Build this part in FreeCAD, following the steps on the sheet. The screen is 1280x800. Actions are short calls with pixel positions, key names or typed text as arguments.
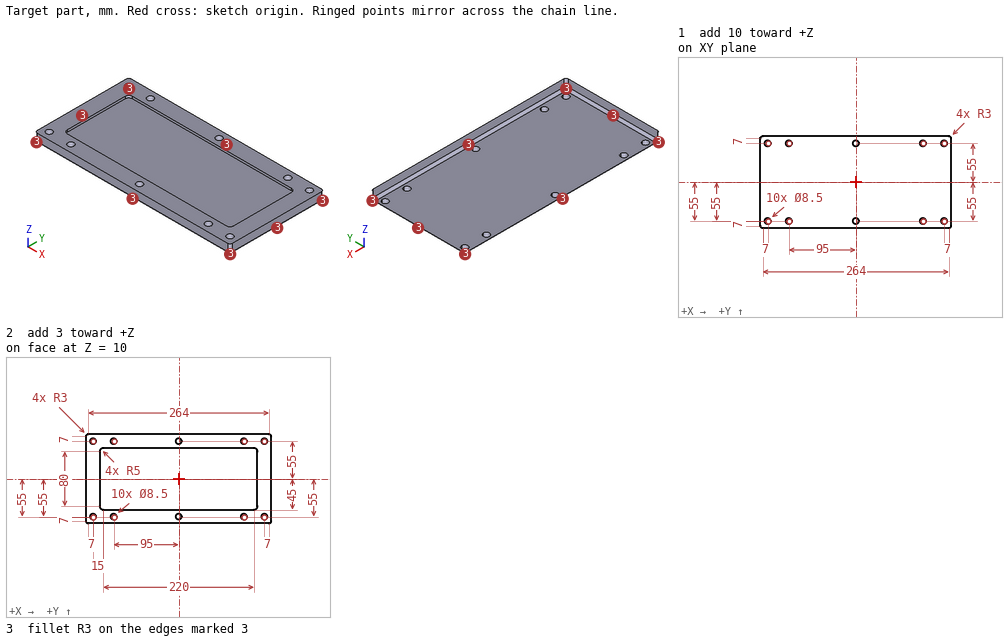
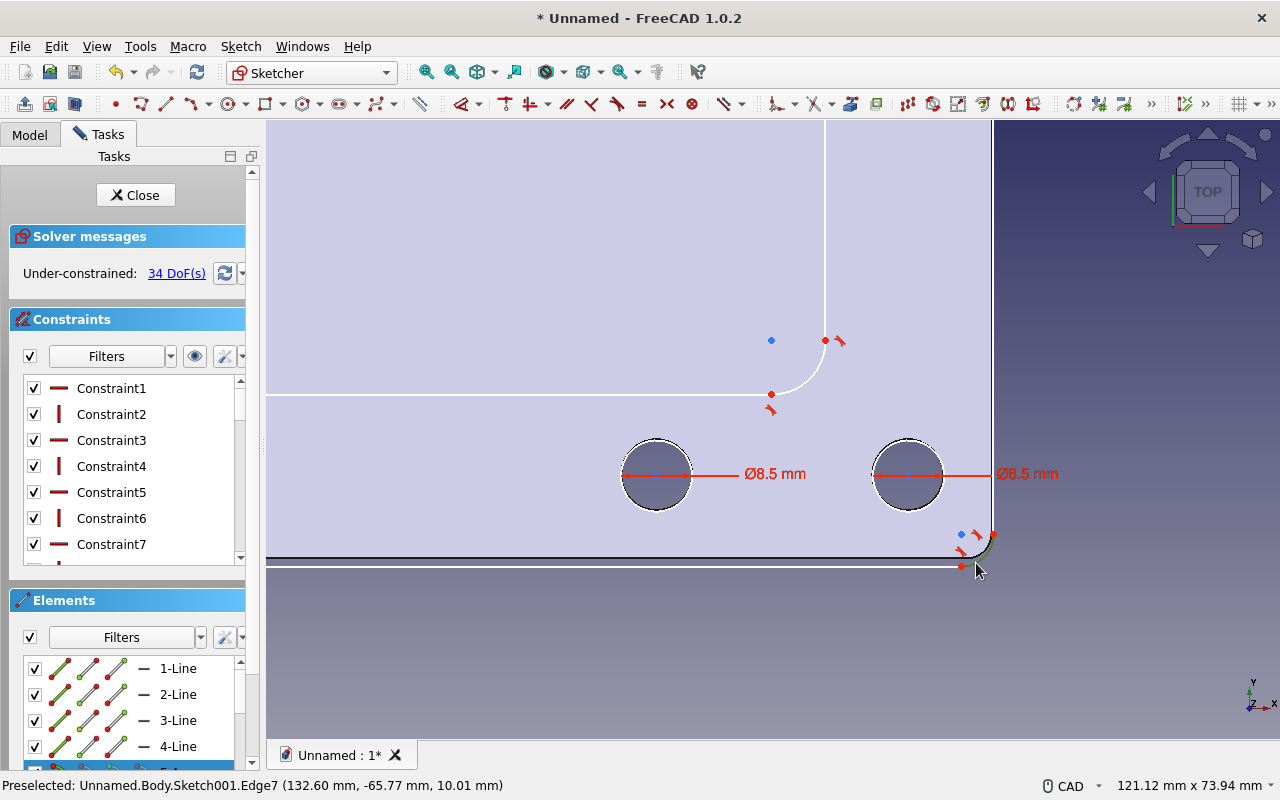
scroll(980, 565, down, 7)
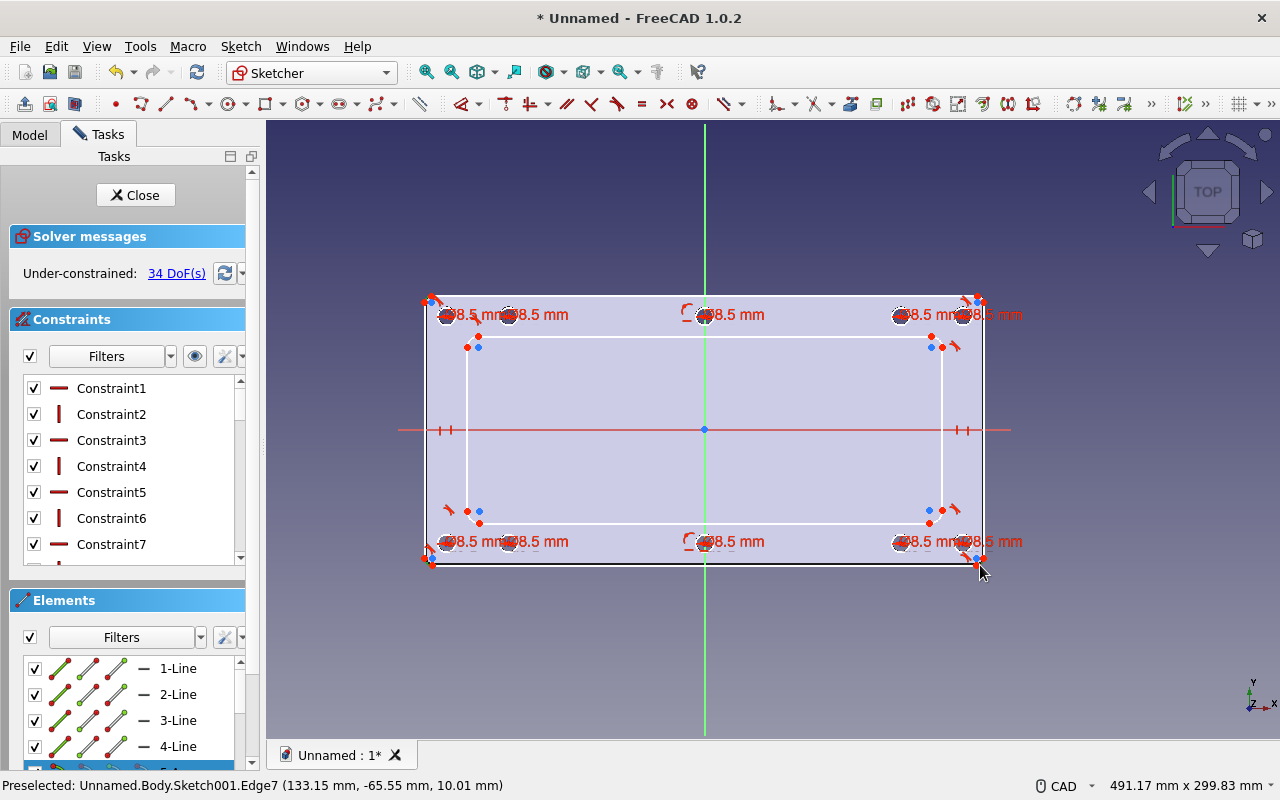
scroll(983, 300, up, 8)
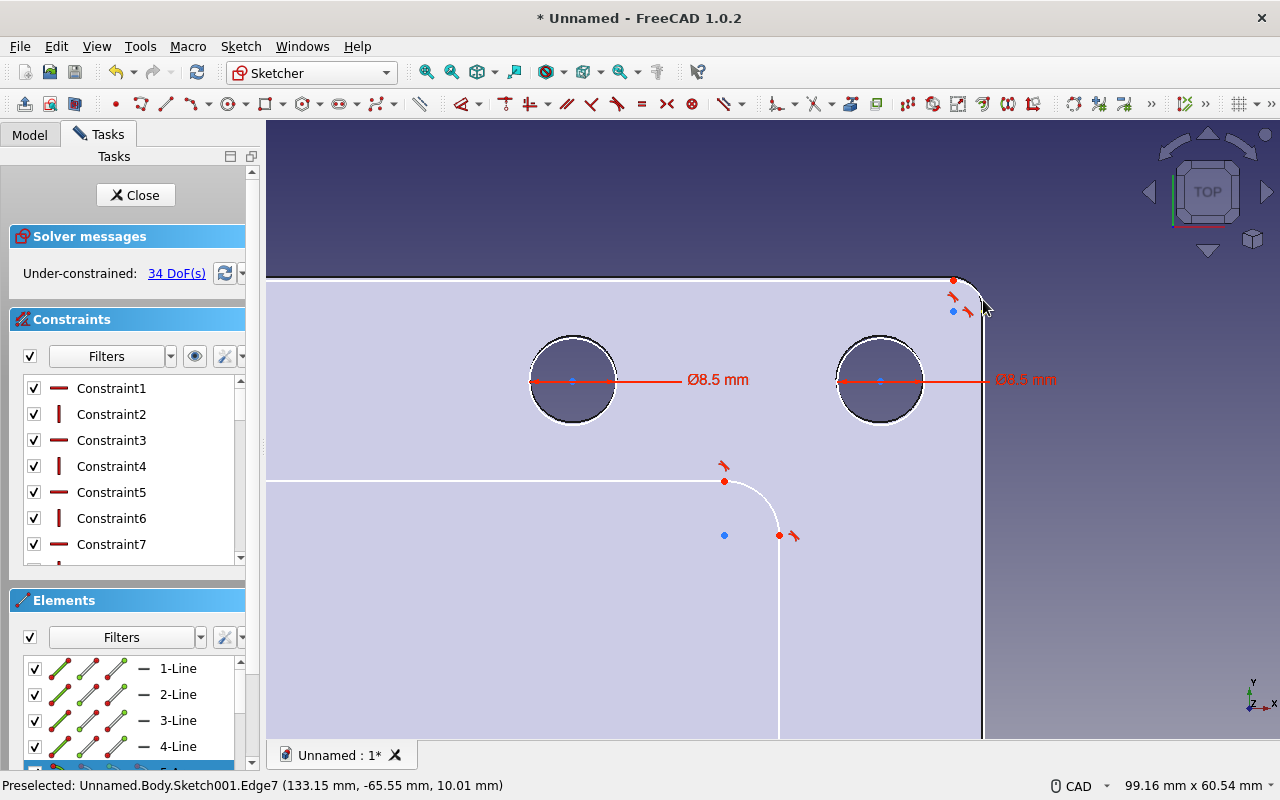
click(981, 297)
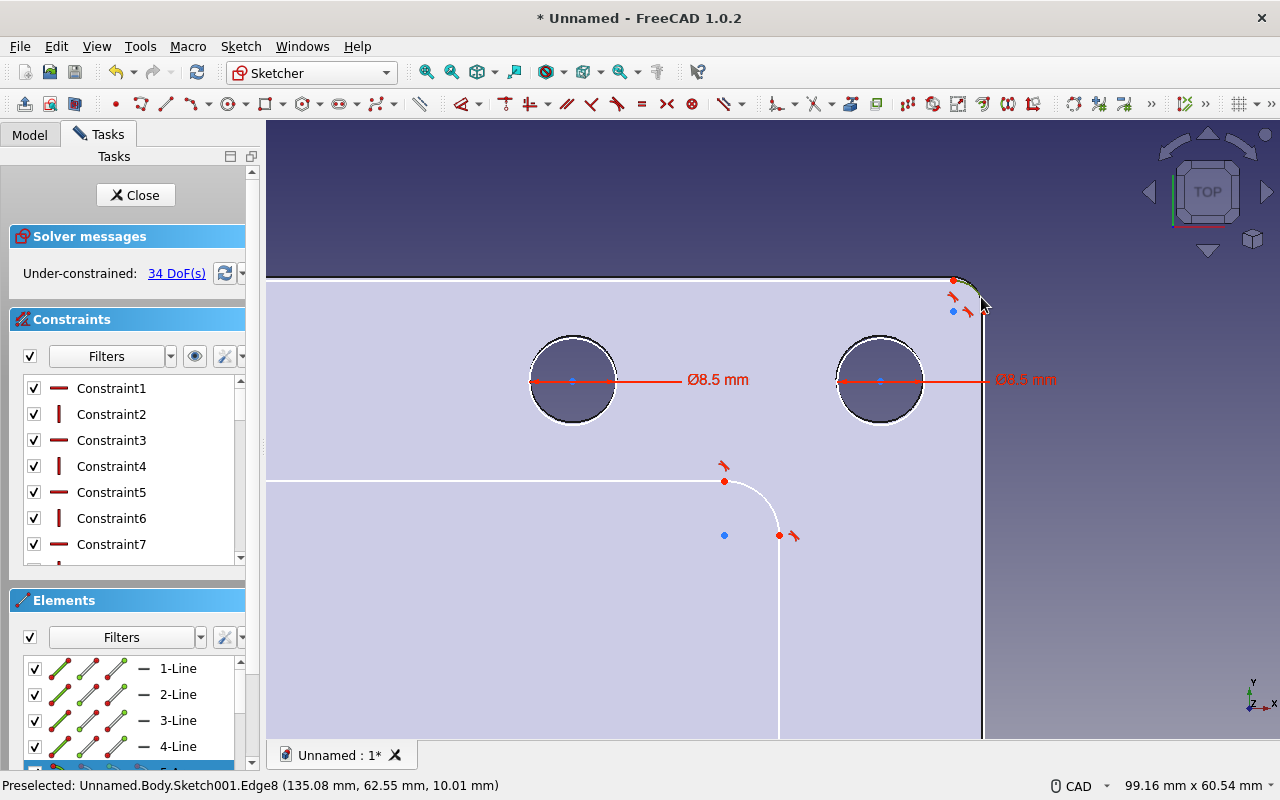
click(642, 104)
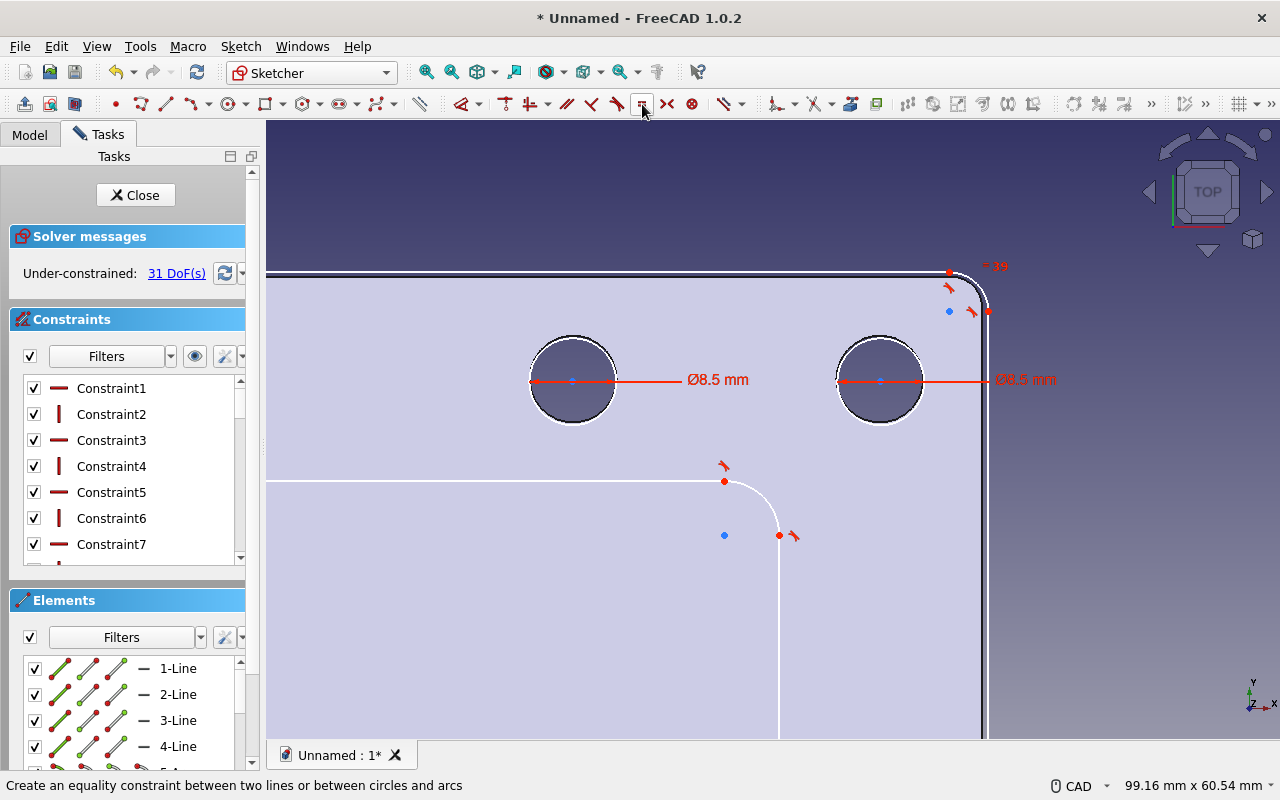
scroll(983, 300, down, 8)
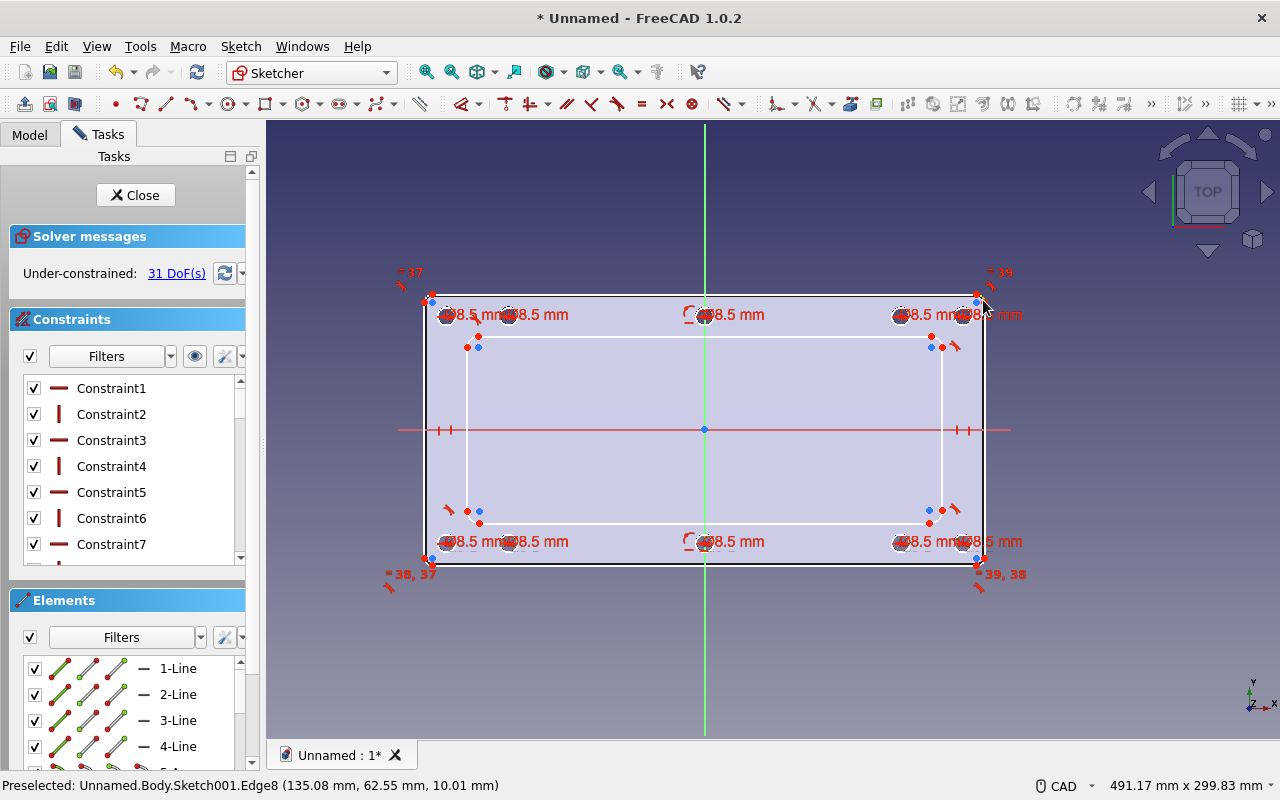
scroll(469, 517, up, 5)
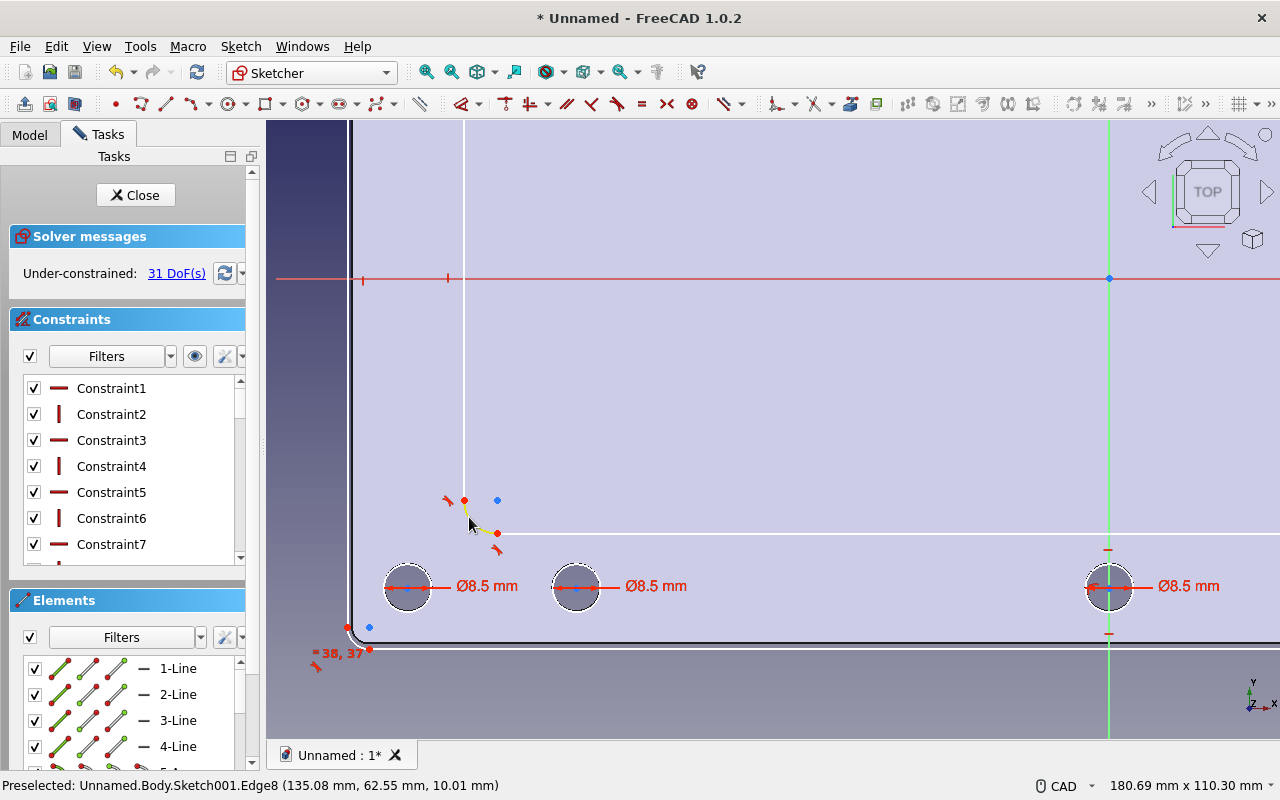
click(468, 516)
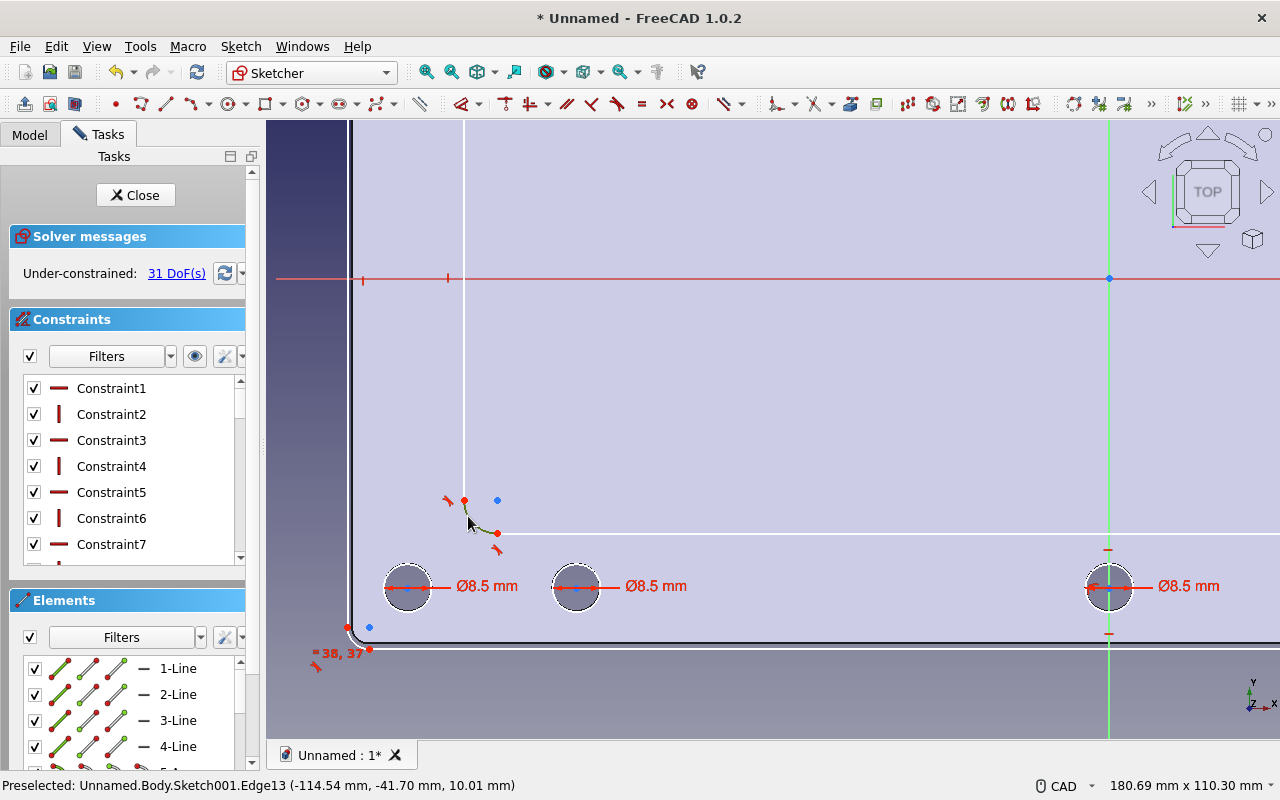
scroll(469, 517, down, 5)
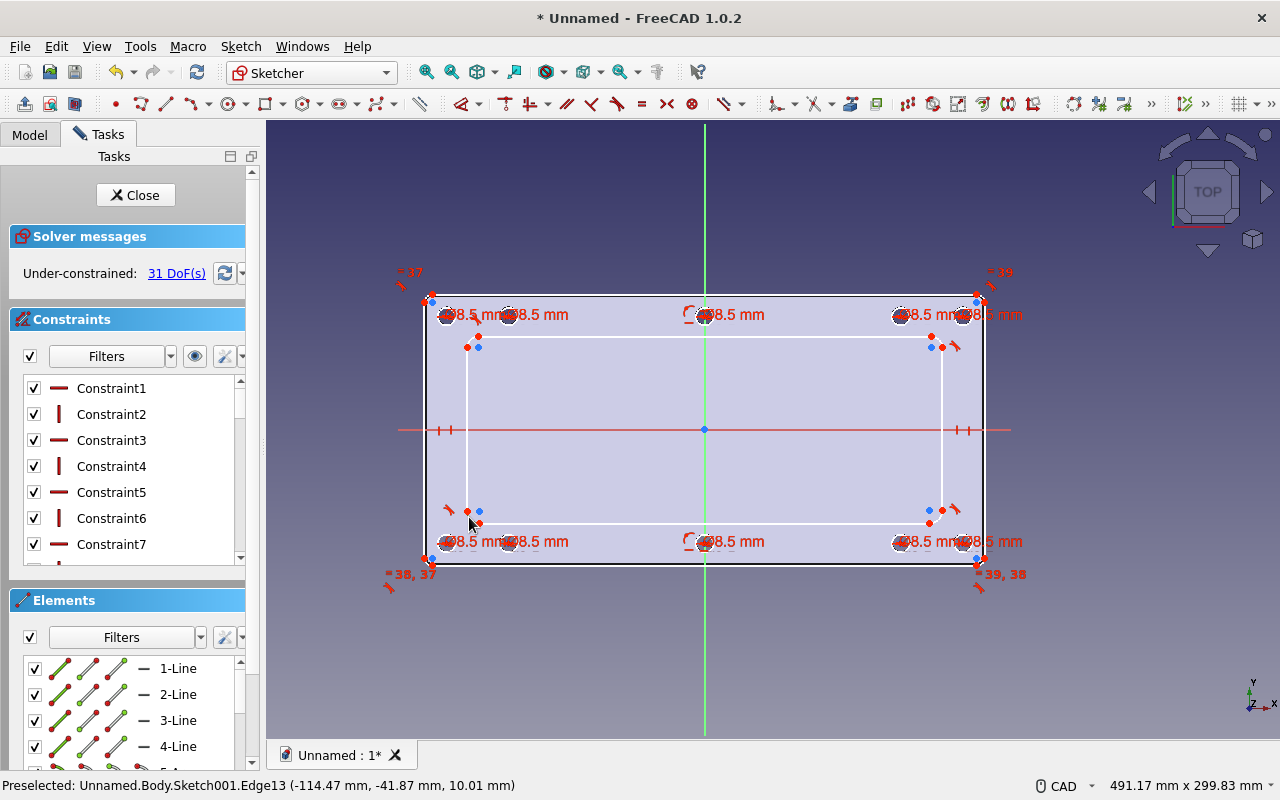
scroll(473, 338, up, 6)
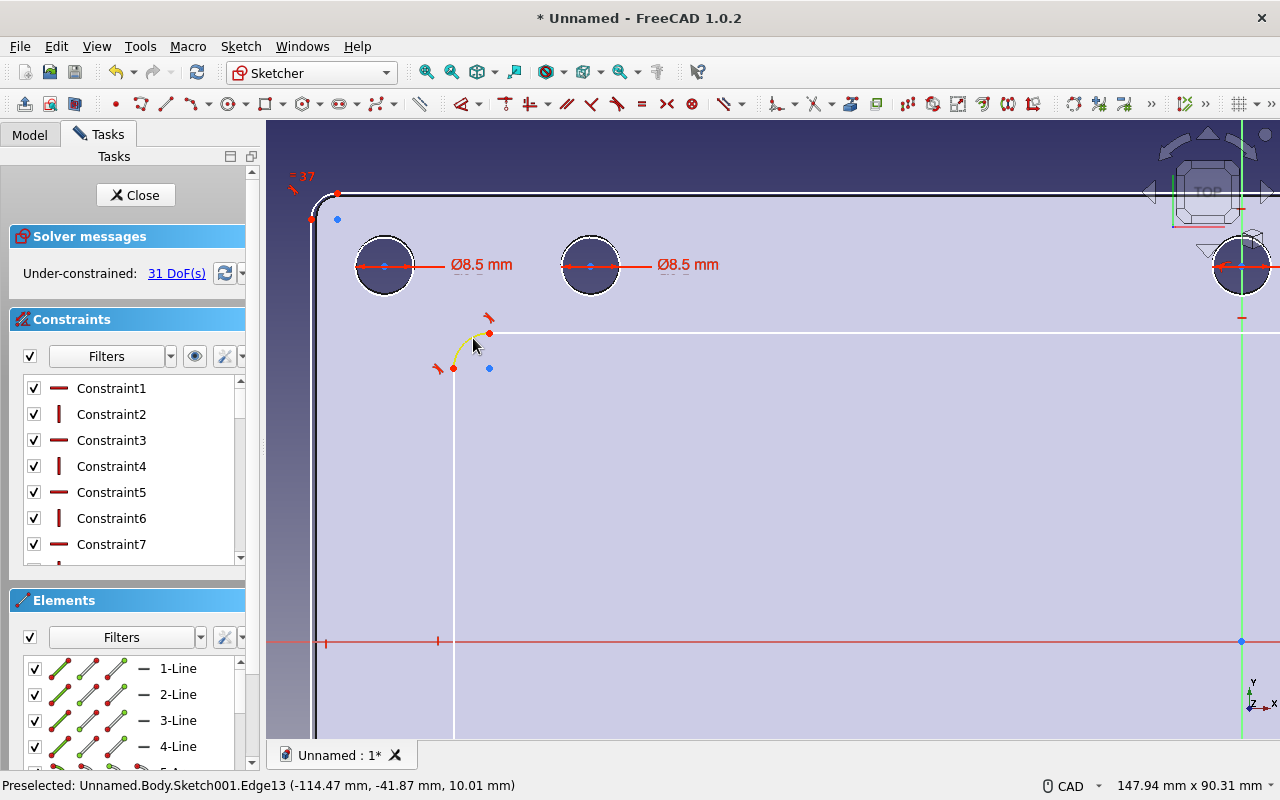
click(473, 337)